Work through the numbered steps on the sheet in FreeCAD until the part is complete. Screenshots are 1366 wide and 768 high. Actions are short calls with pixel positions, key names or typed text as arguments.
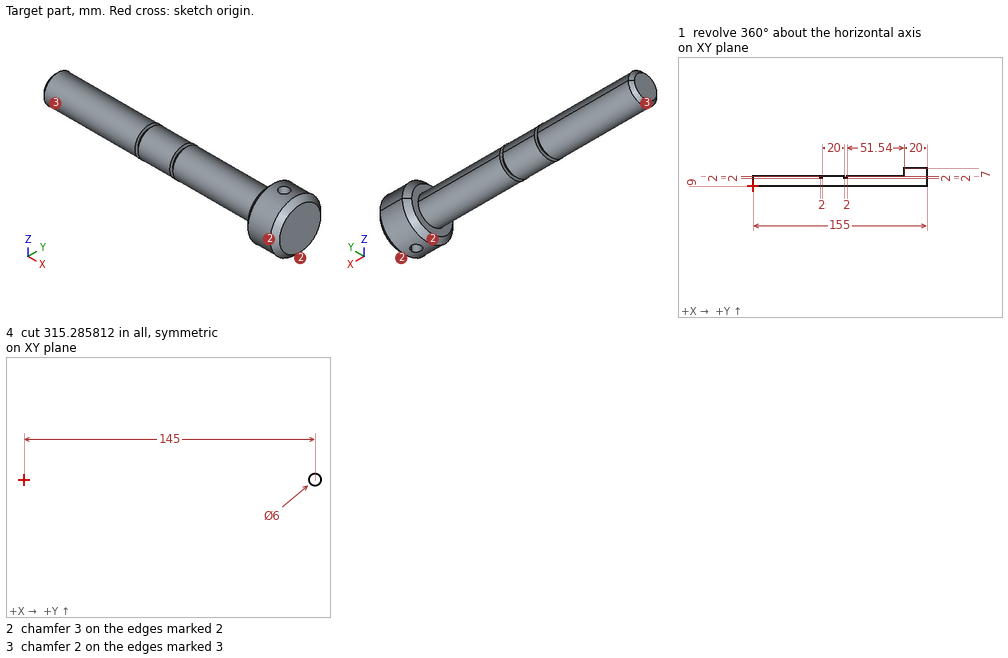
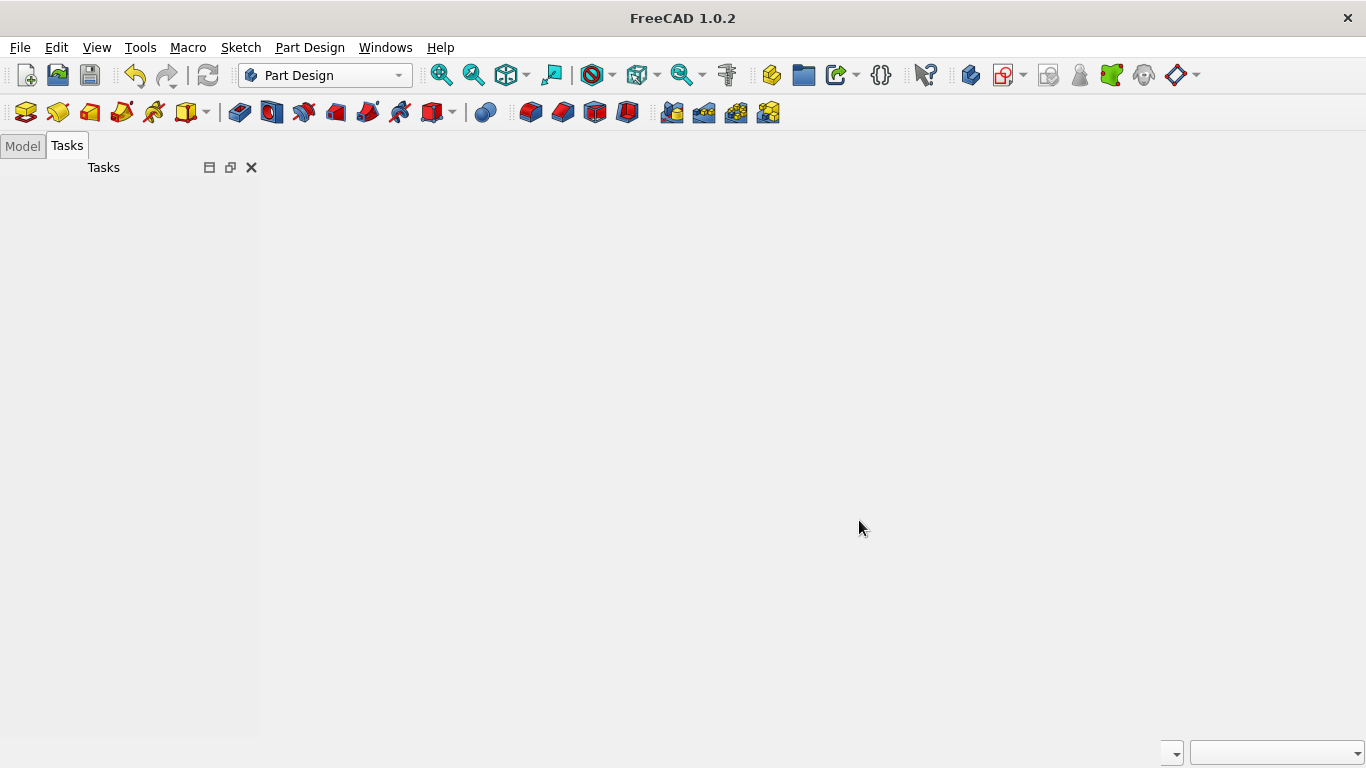
click(26, 76)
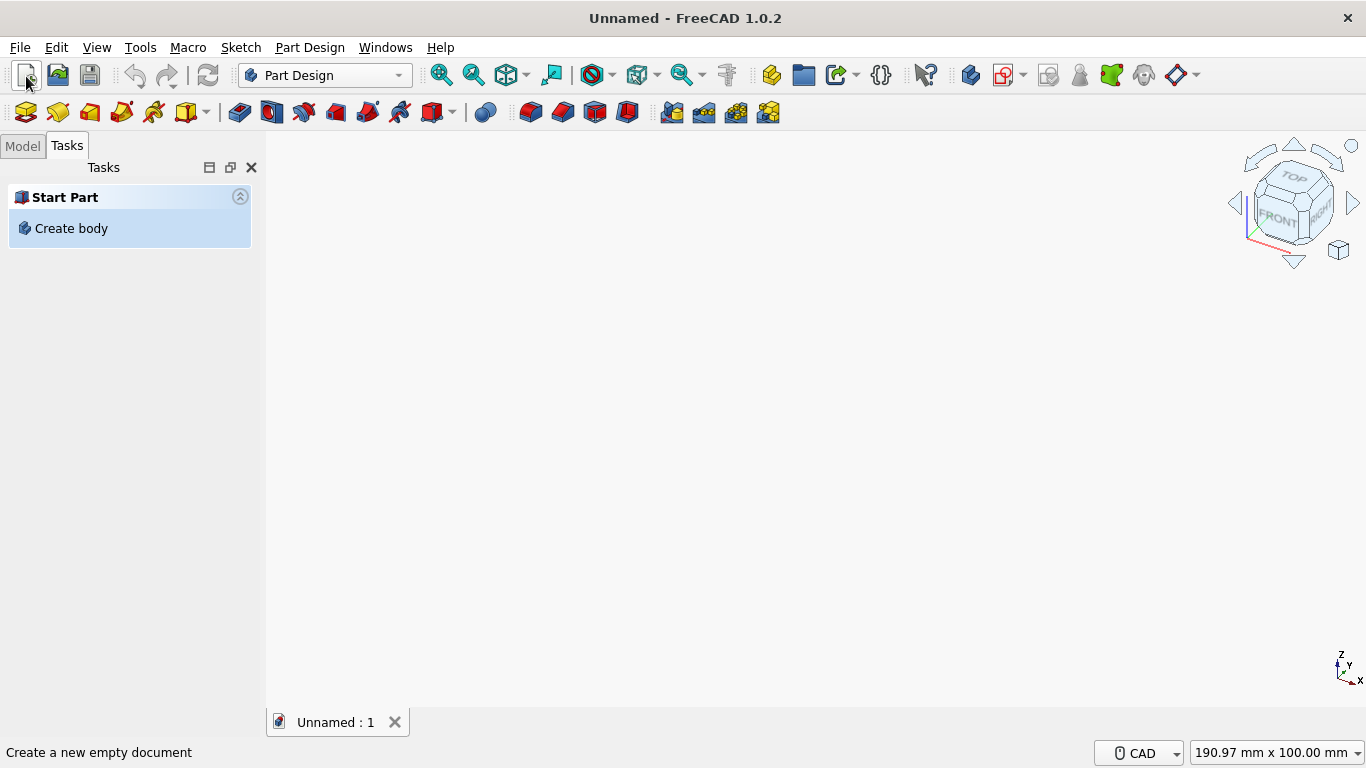
click(1004, 76)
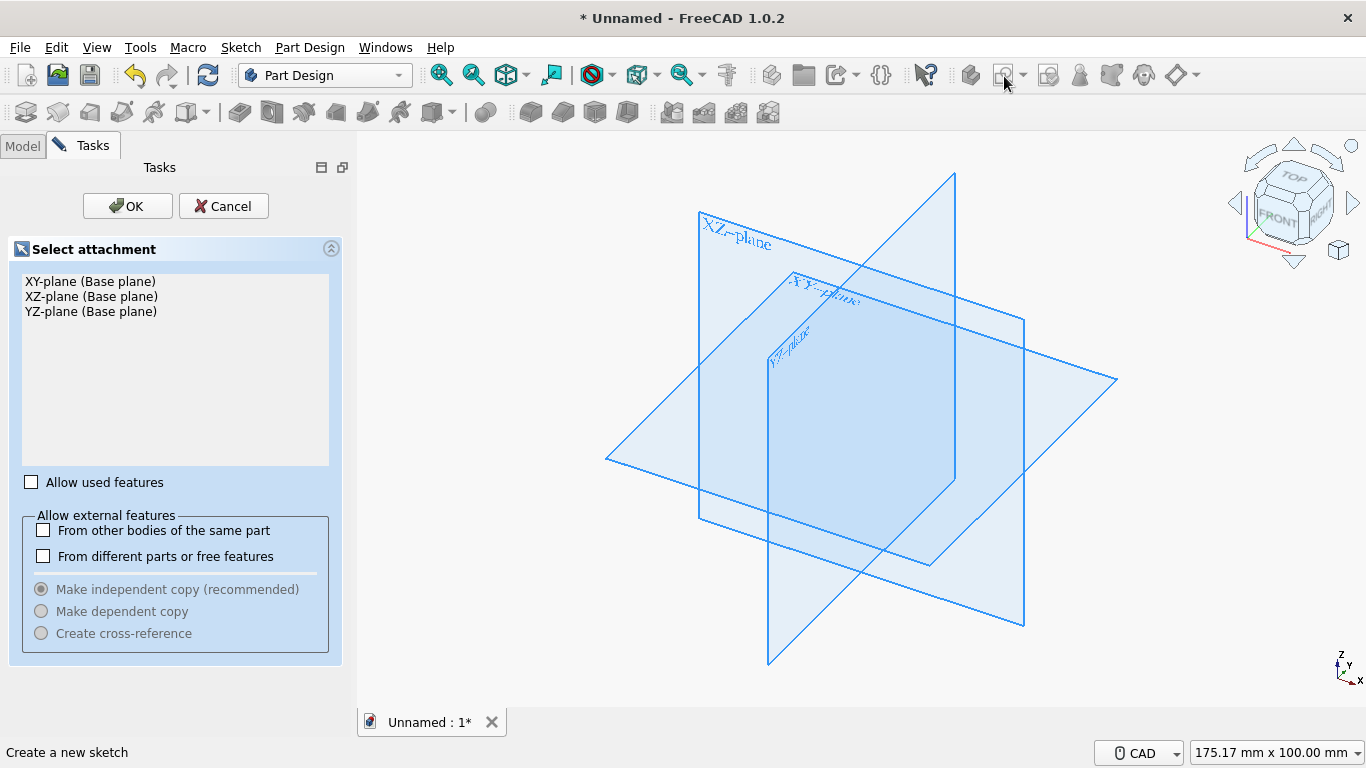
click(82, 282)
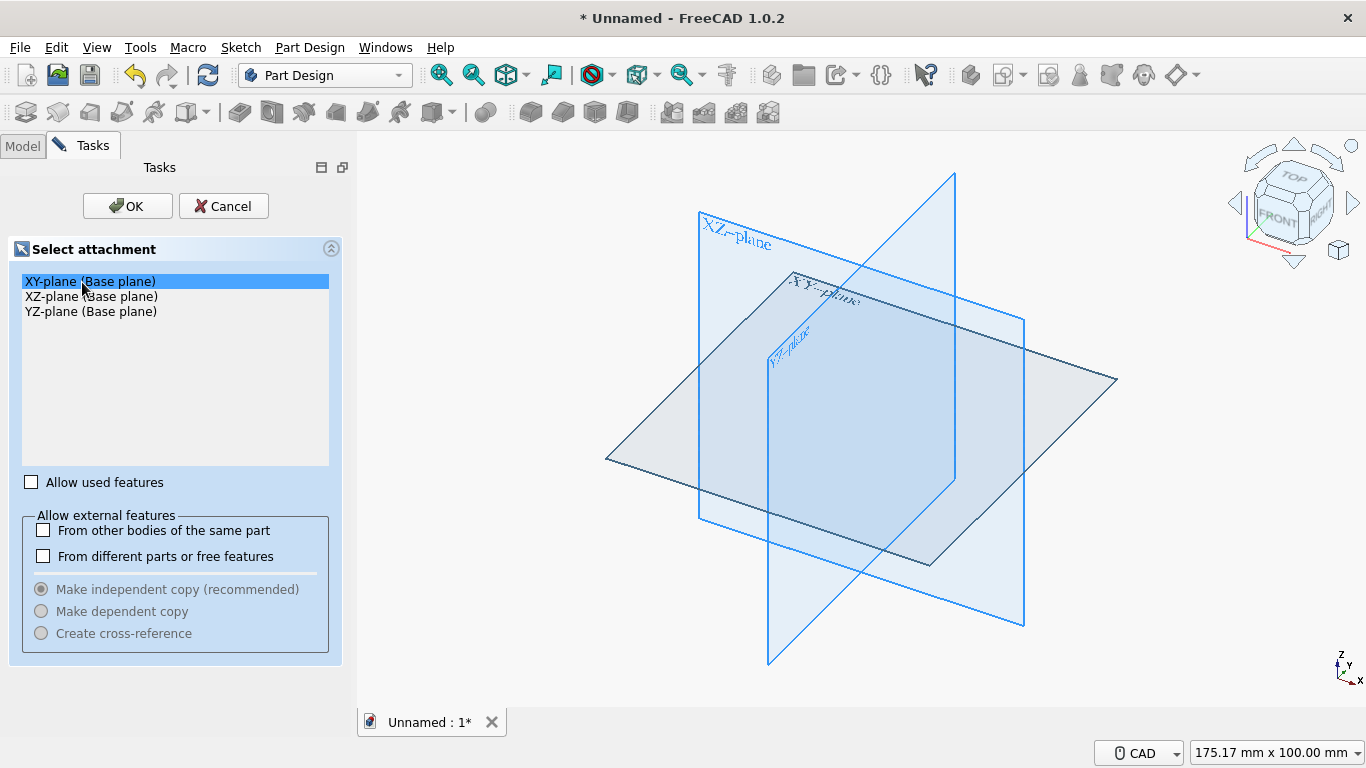
click(128, 206)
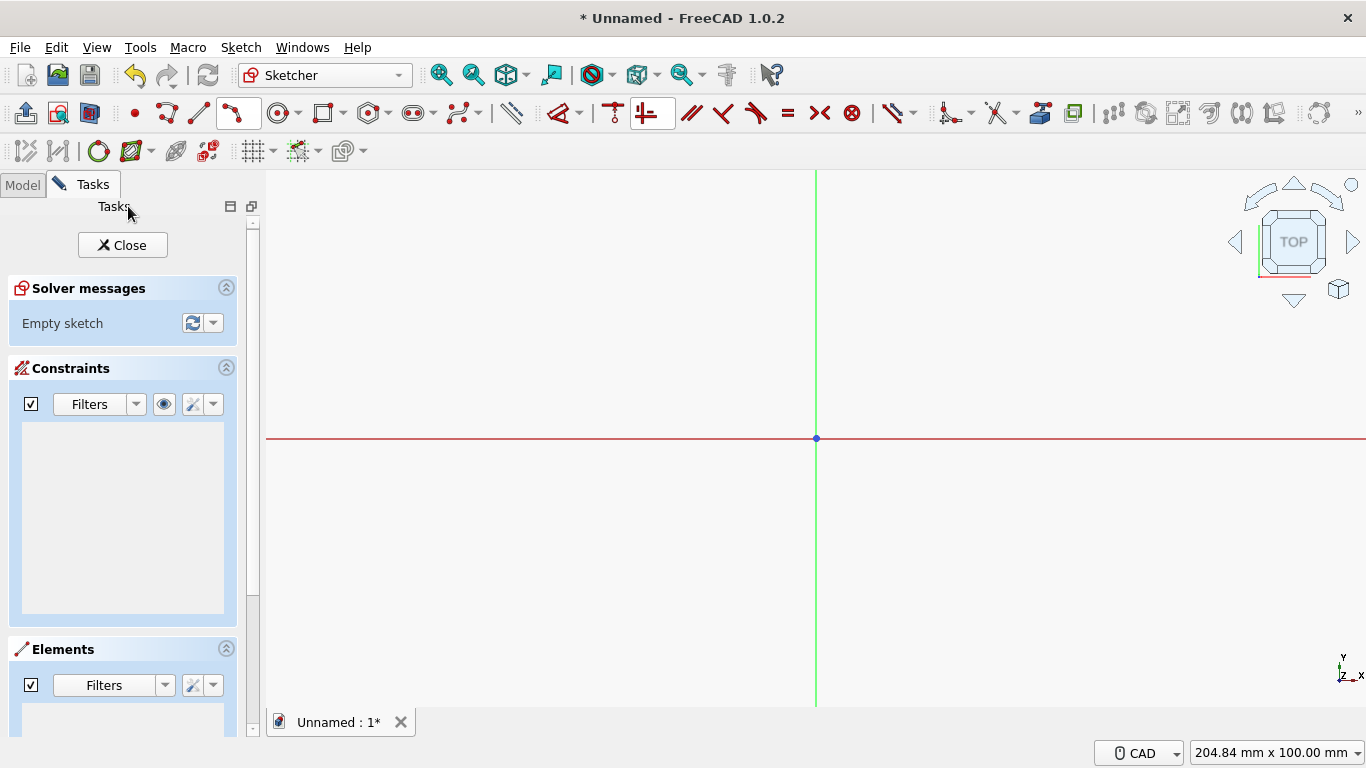
scroll(294, 491, down, 3)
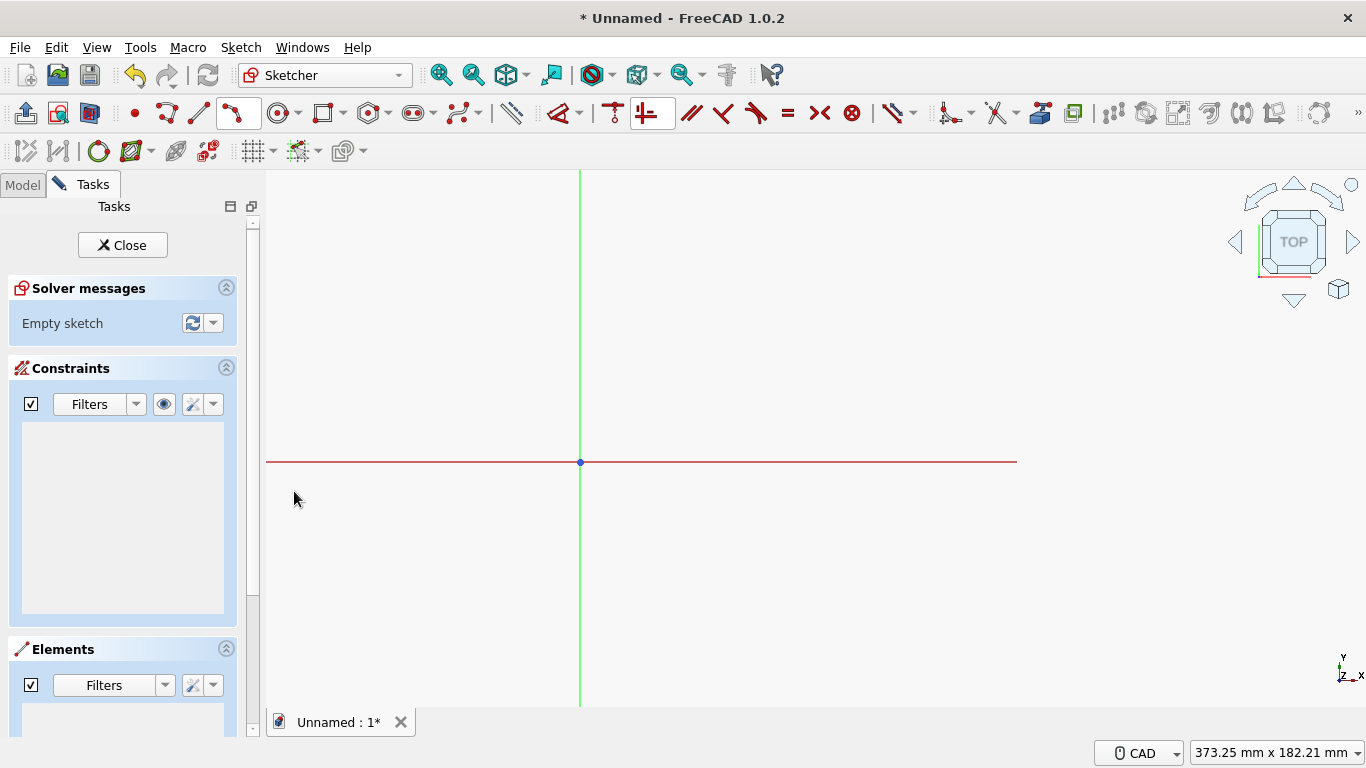
scroll(934, 440, up, 2)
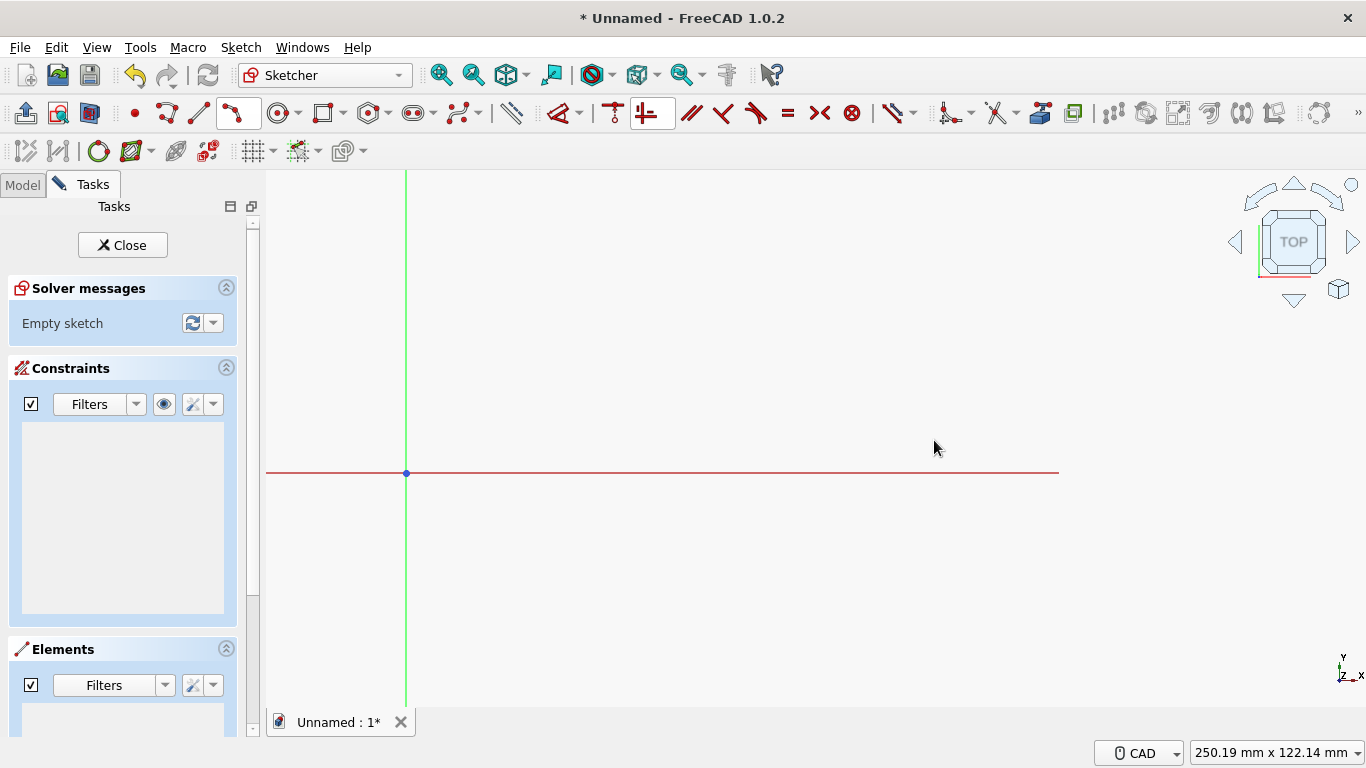
click(168, 114)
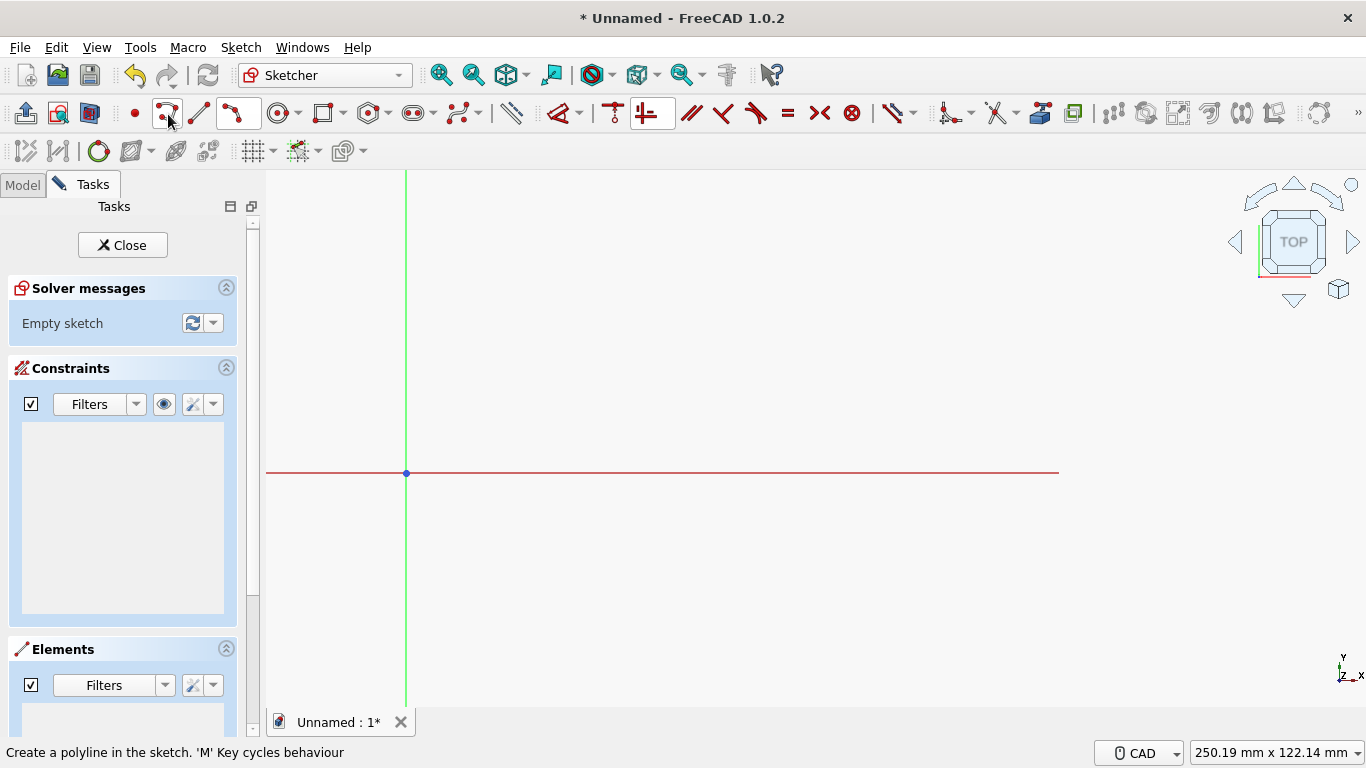
click(406, 473)
click(1088, 464)
click(1088, 403)
click(1000, 403)
click(1000, 434)
click(773, 434)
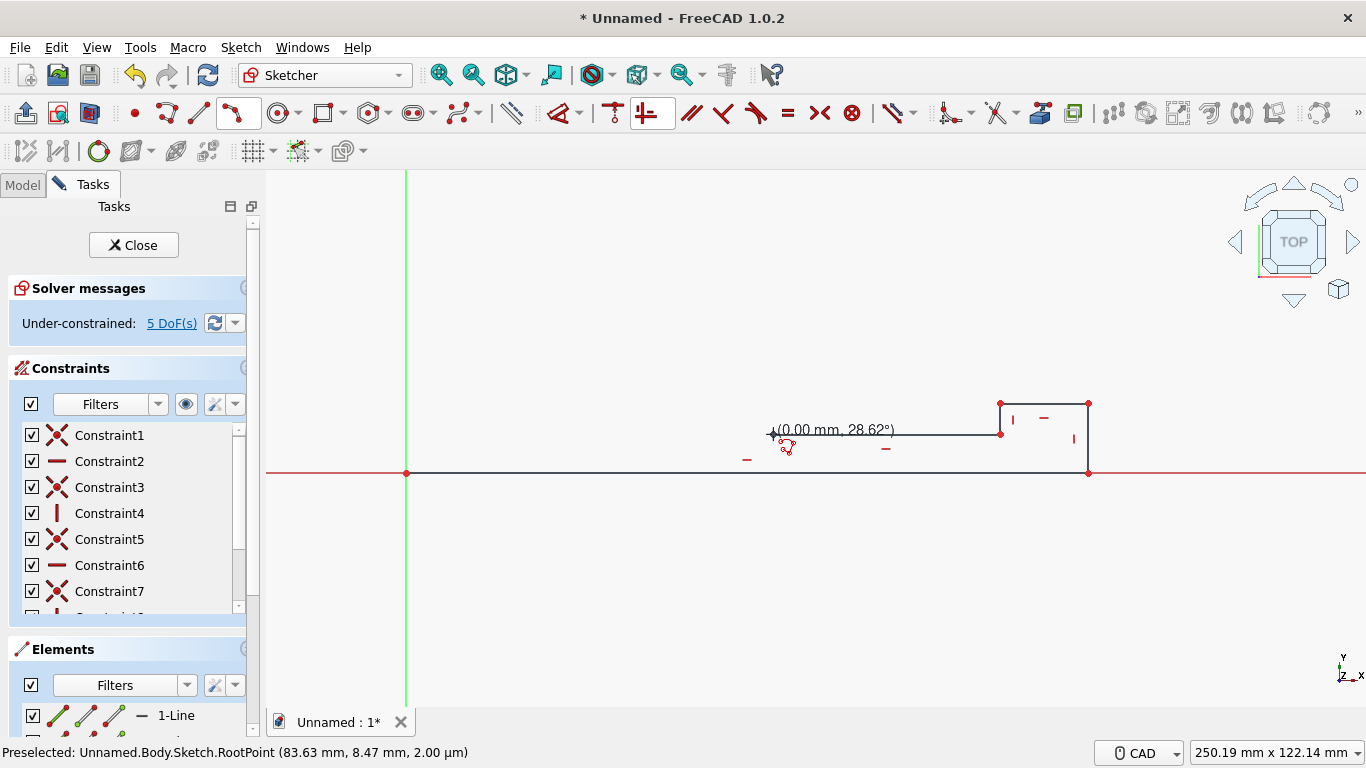
scroll(773, 442, up, 3)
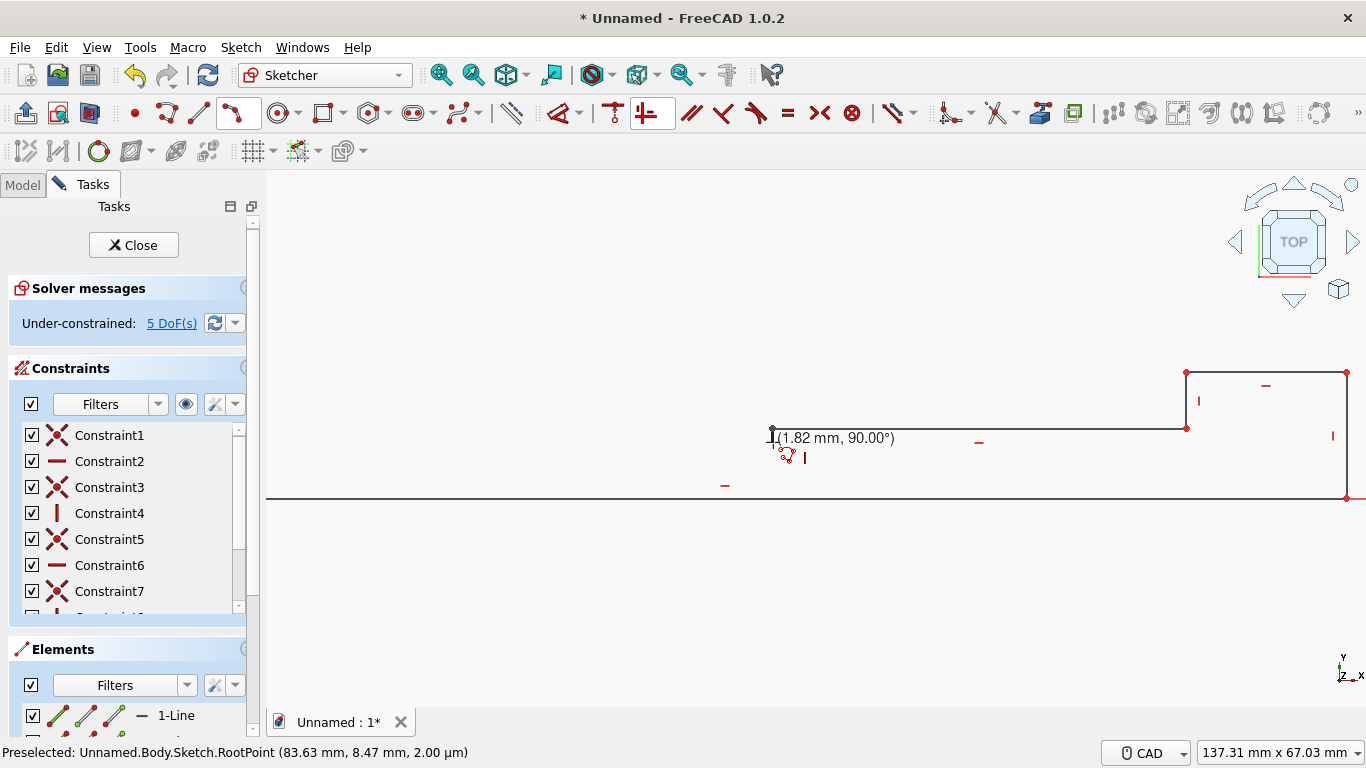
click(773, 442)
click(757, 442)
click(757, 426)
click(597, 426)
click(597, 442)
click(581, 442)
click(581, 426)